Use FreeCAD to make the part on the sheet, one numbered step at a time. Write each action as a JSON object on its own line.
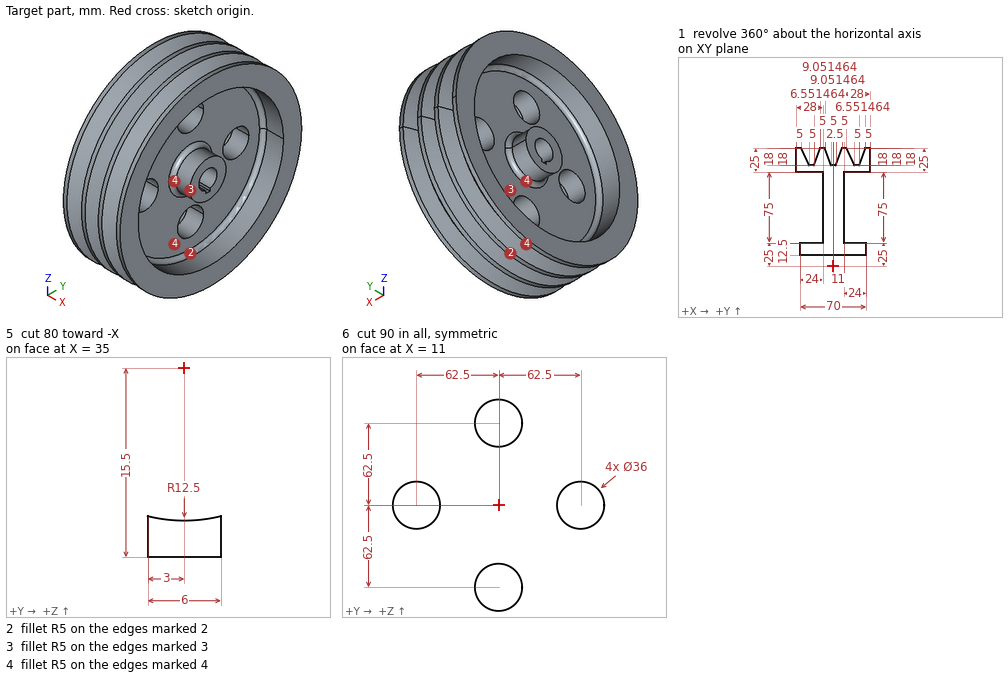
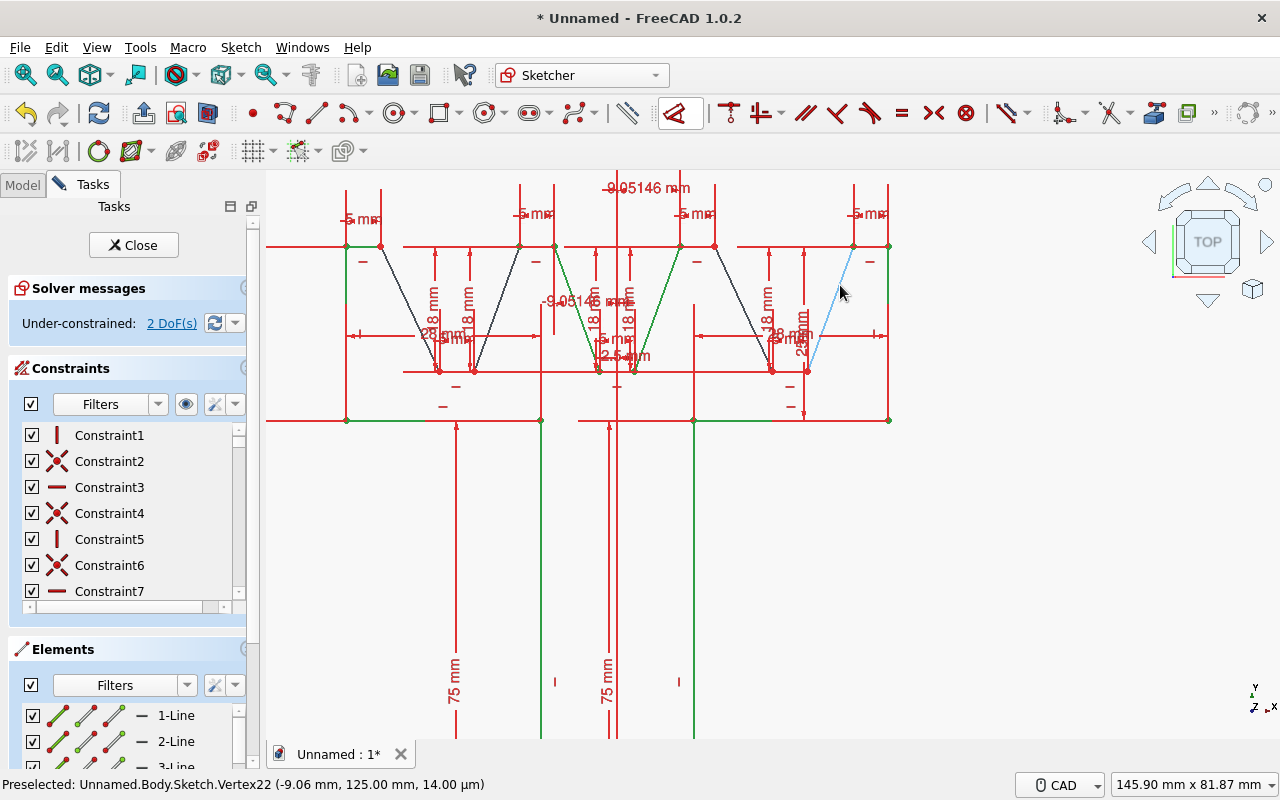
{"action": "left_click", "coordinate": [840, 284]}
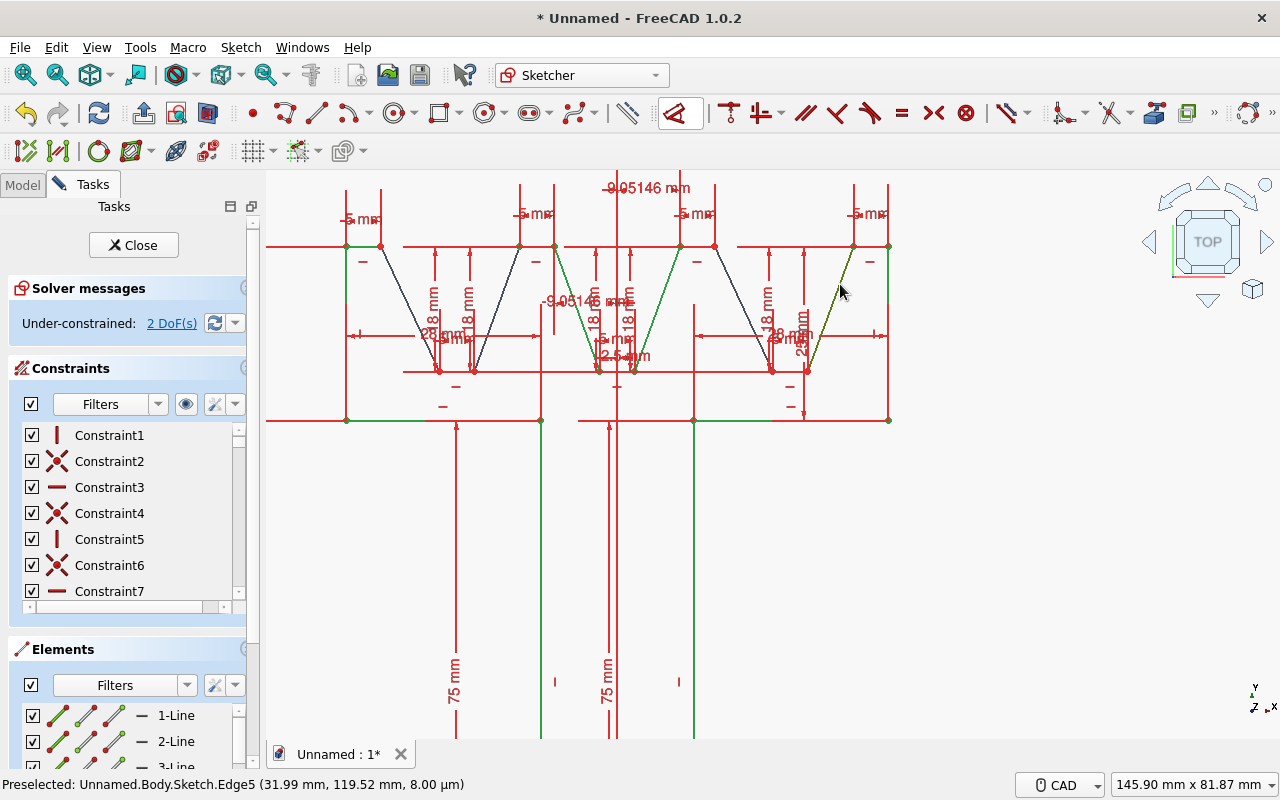
{"action": "left_click", "coordinate": [698, 114]}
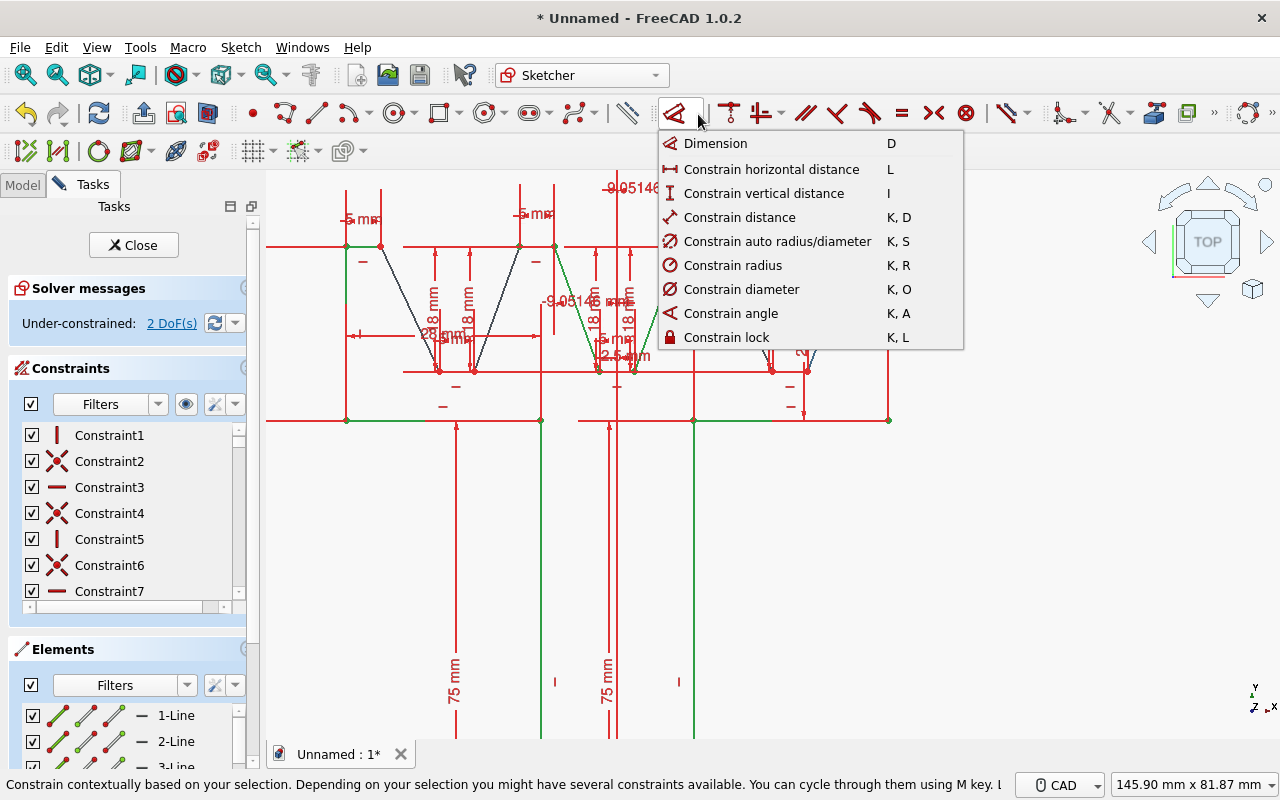
{"action": "left_click", "coordinate": [811, 169]}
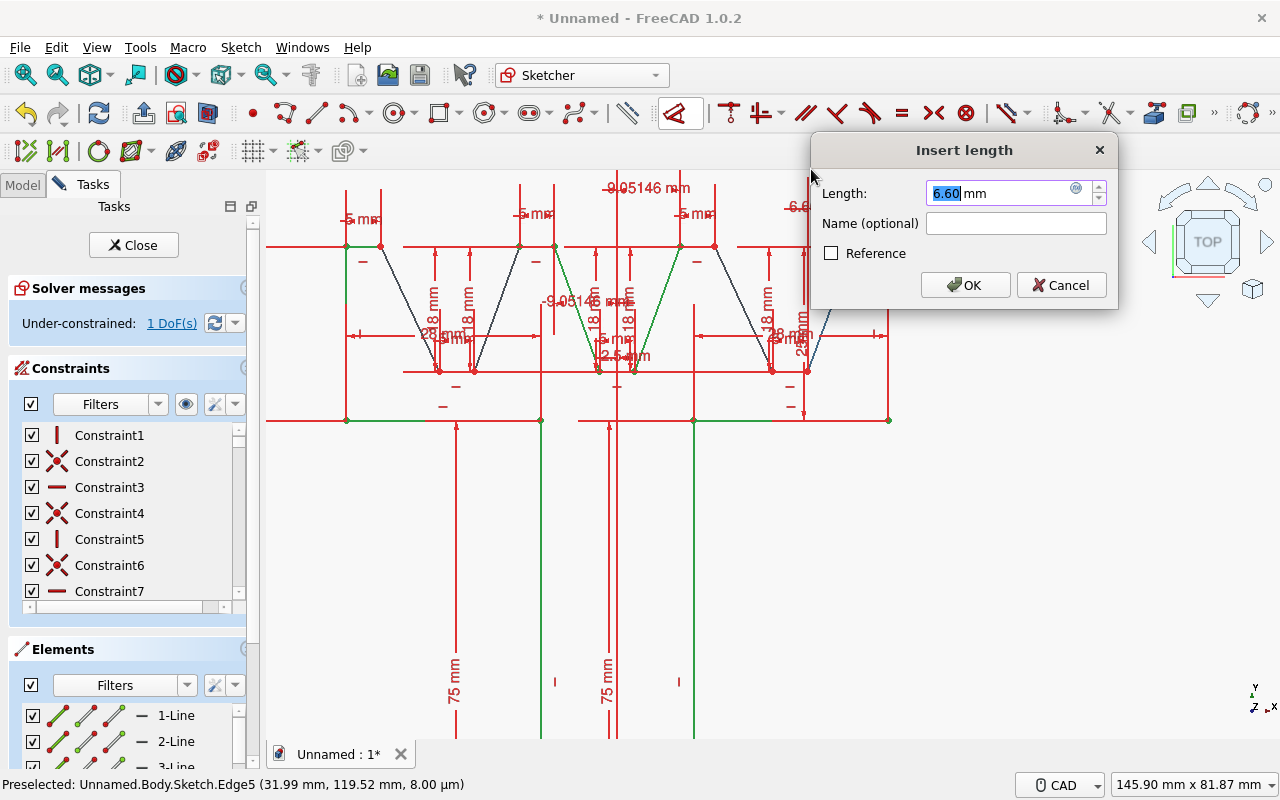
{"action": "type", "text": "6.551464"}
{"action": "key", "text": "Return"}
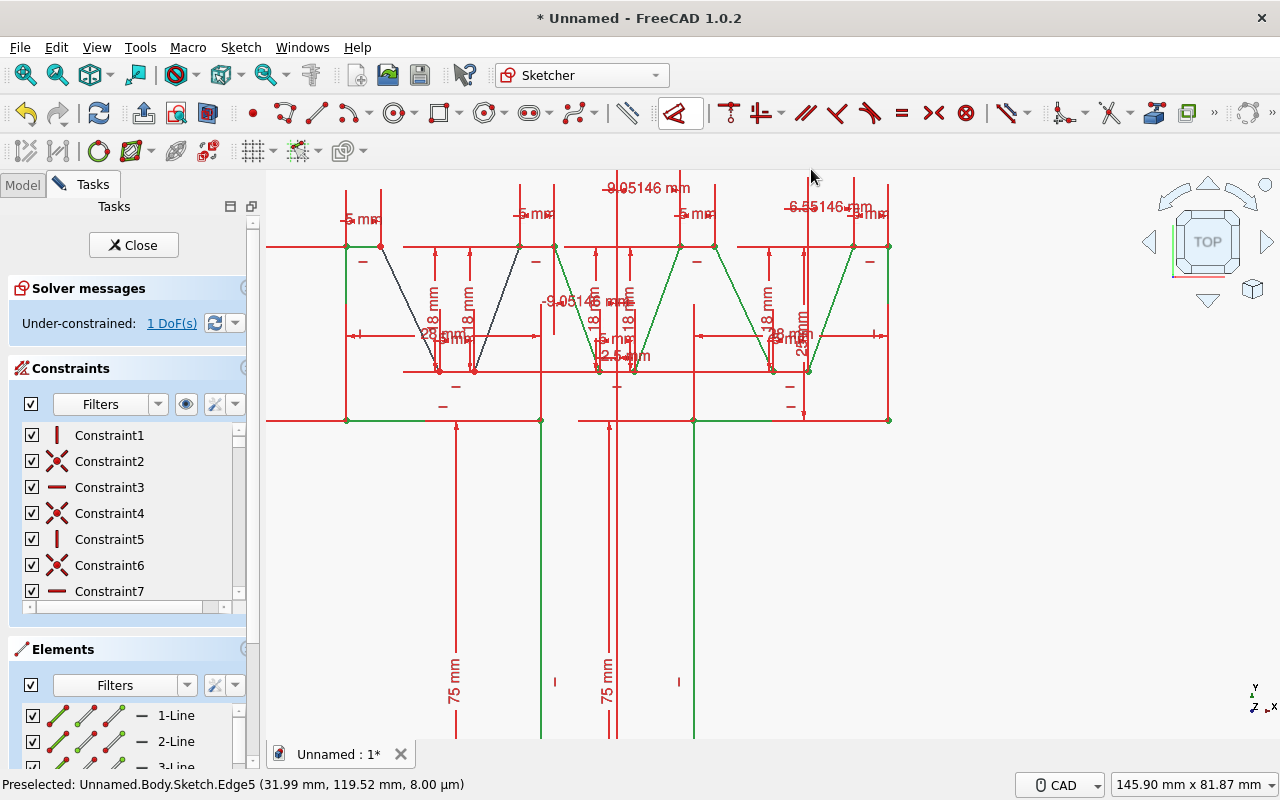
{"action": "left_click", "coordinate": [506, 284]}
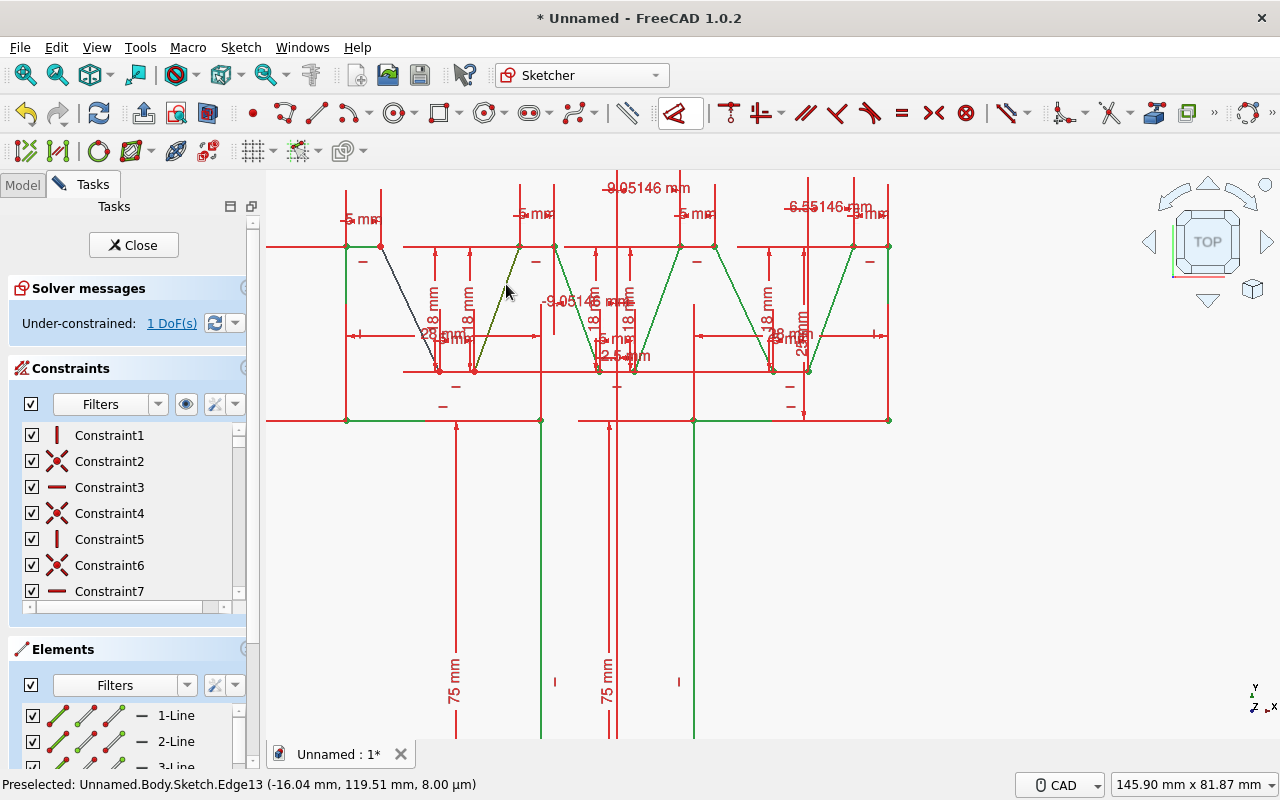
{"action": "left_click", "coordinate": [698, 114]}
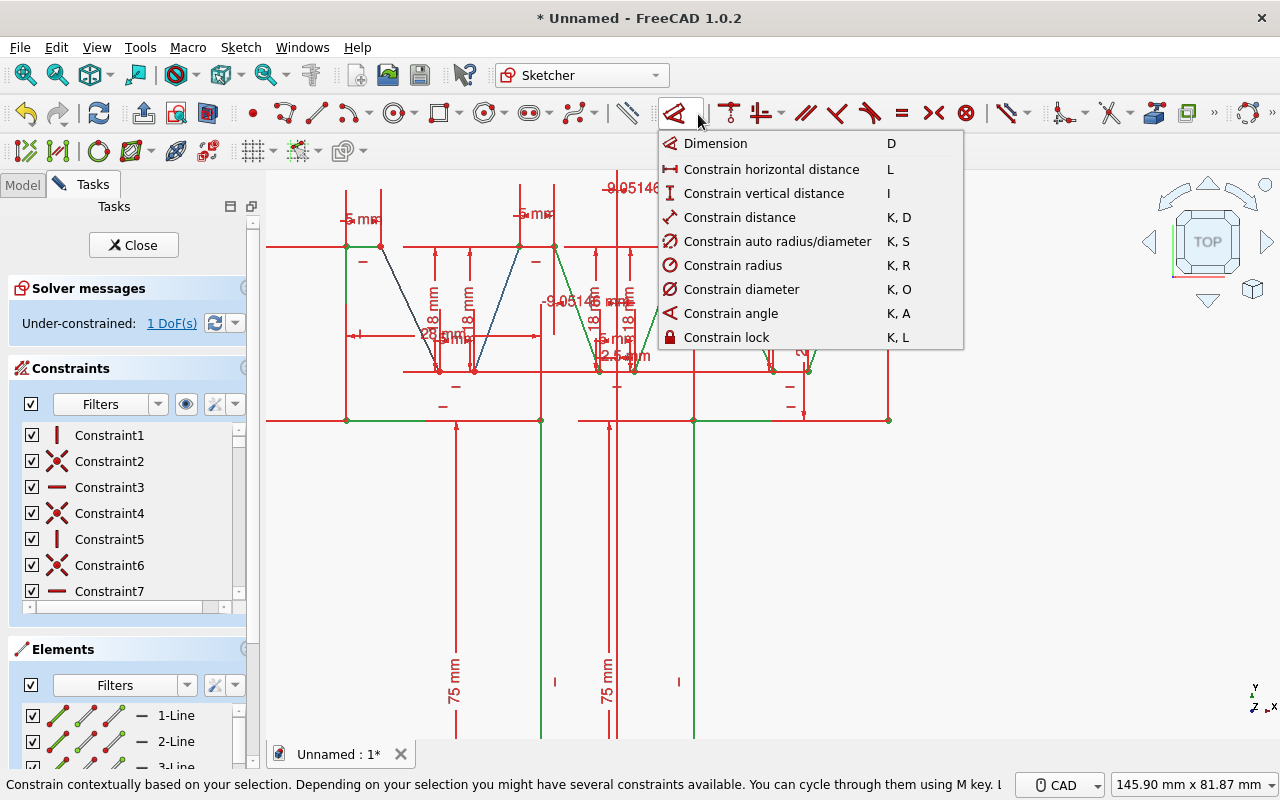
{"action": "left_click", "coordinate": [811, 169]}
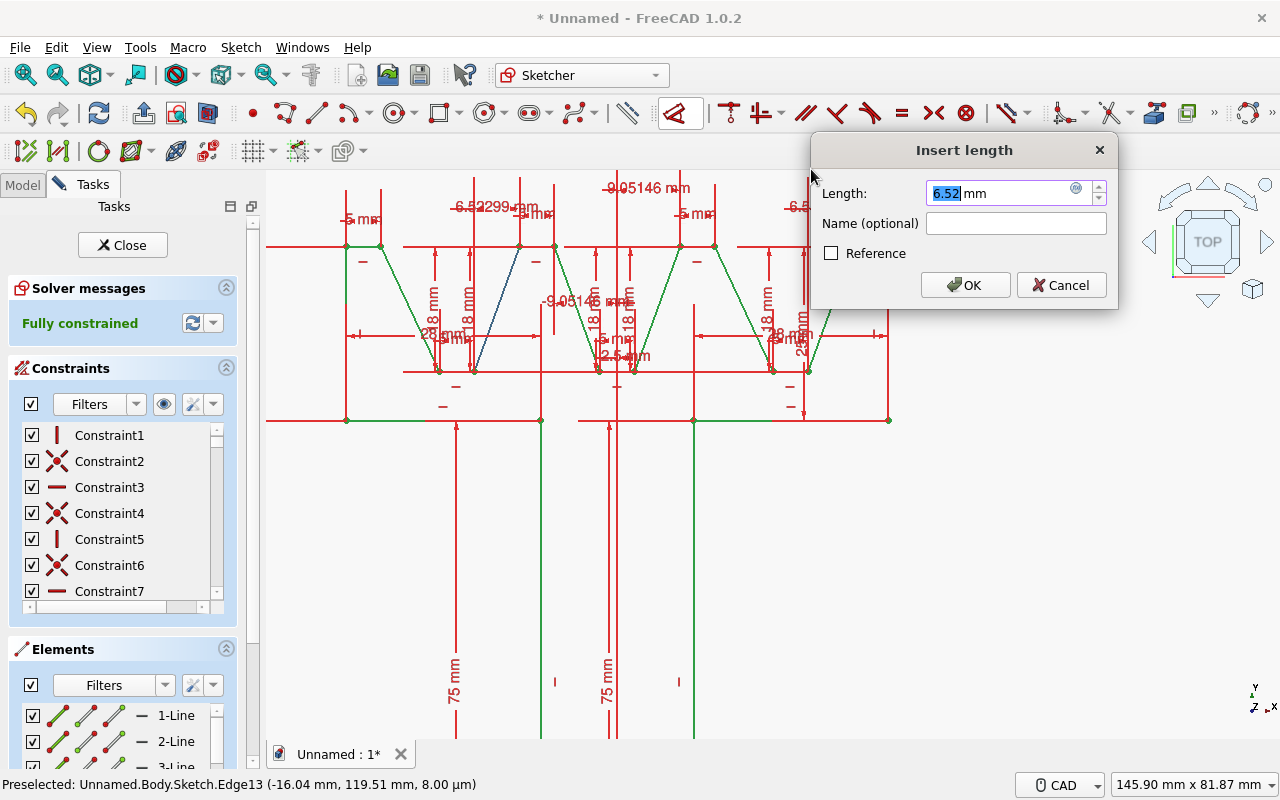
{"action": "type", "text": "6.551464"}
{"action": "key", "text": "Return"}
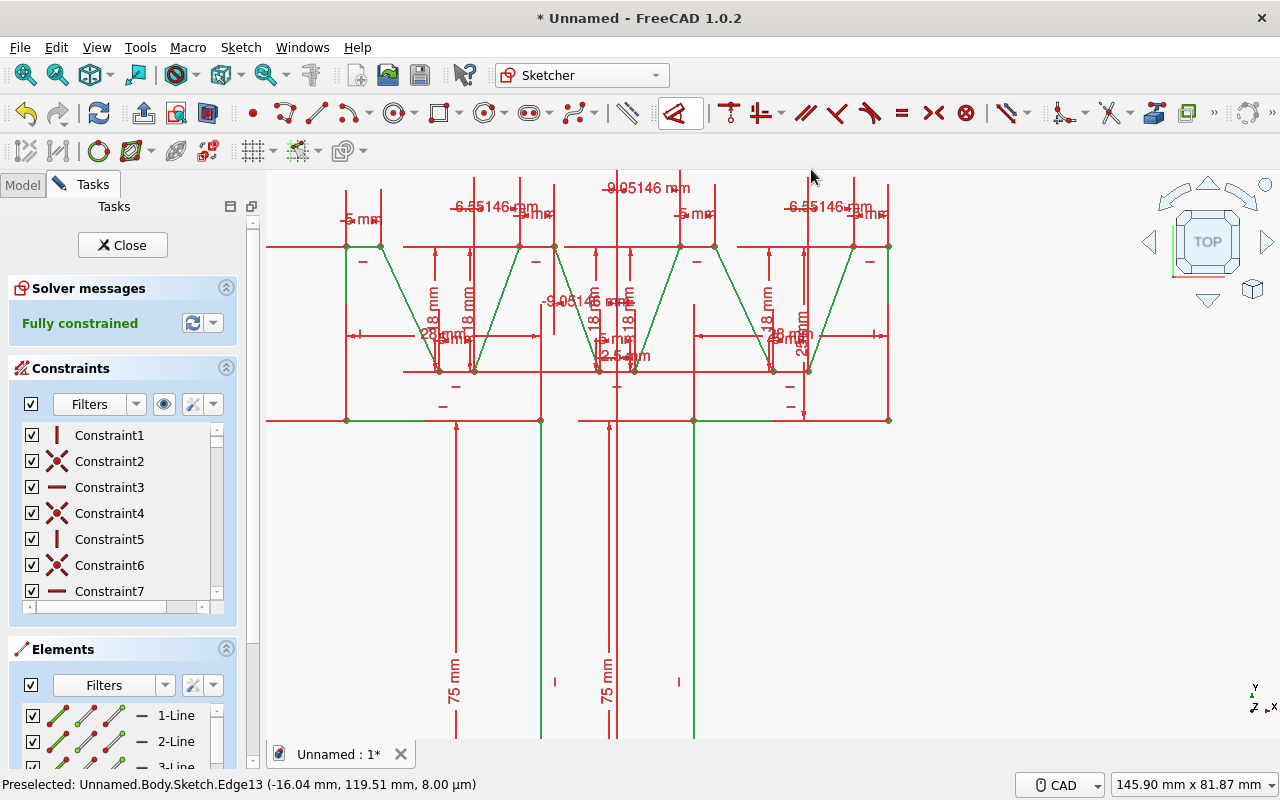
{"action": "left_click", "coordinate": [123, 245]}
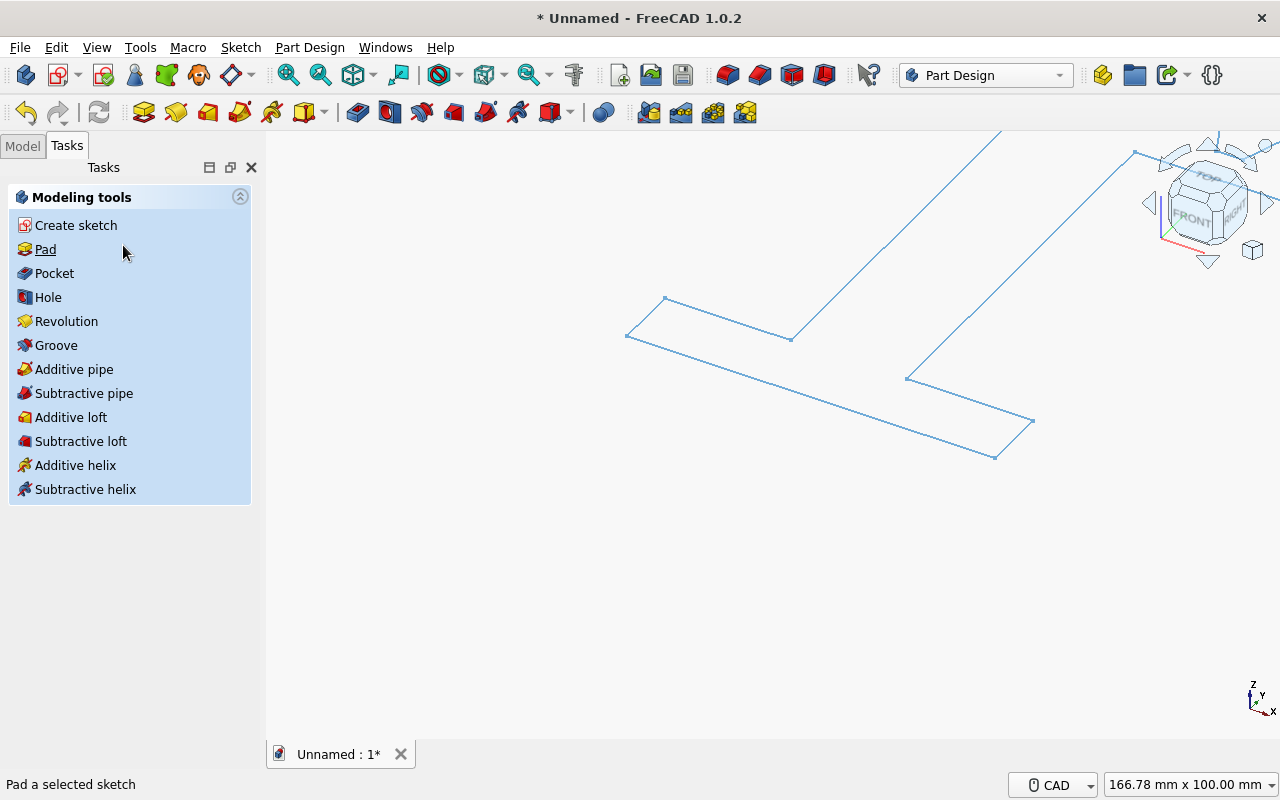
{"action": "left_click", "coordinate": [176, 112]}